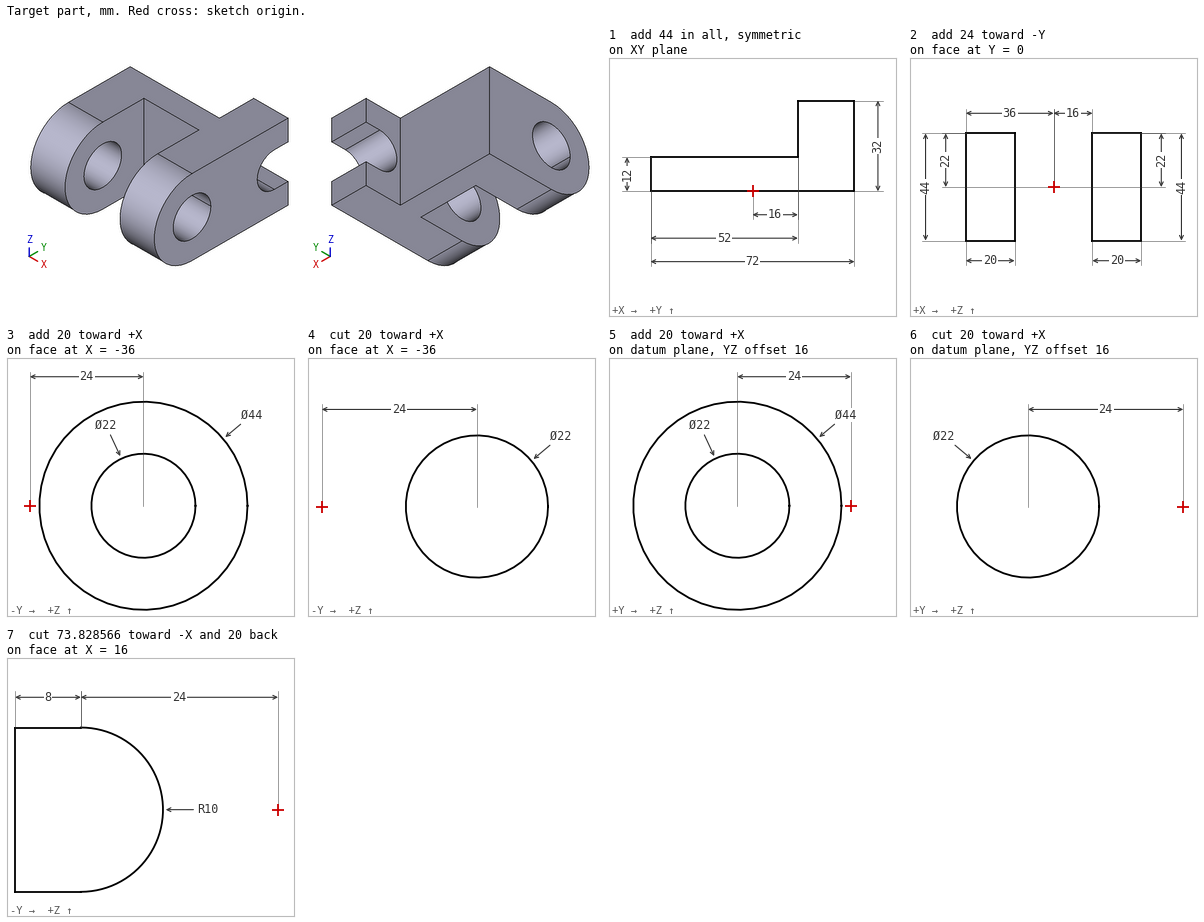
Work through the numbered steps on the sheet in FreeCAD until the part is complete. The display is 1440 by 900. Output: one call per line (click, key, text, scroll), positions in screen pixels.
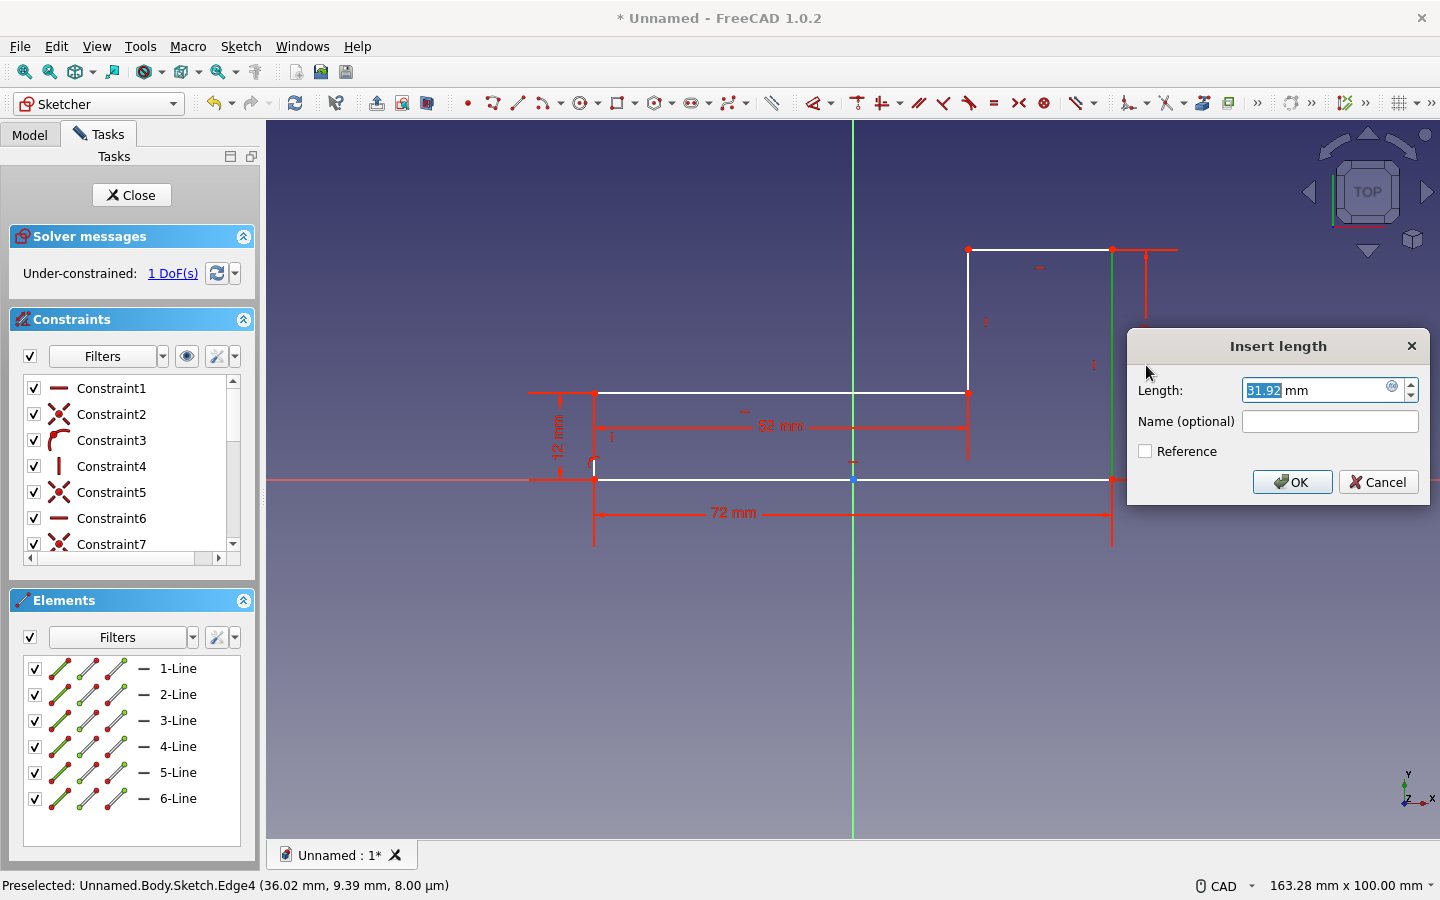
text(32)
key(Return)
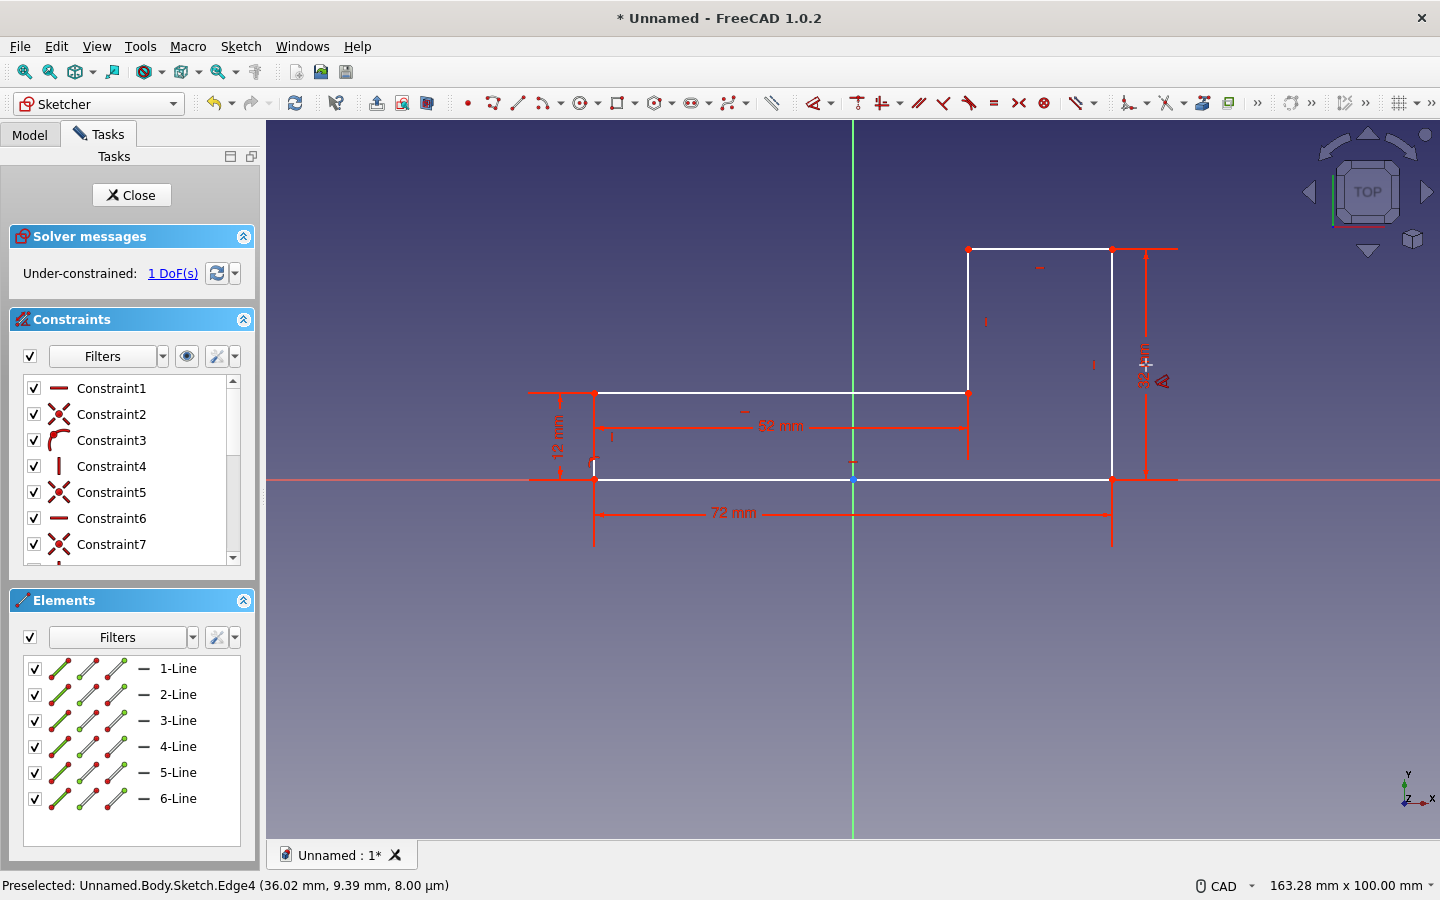
click(968, 393)
click(911, 514)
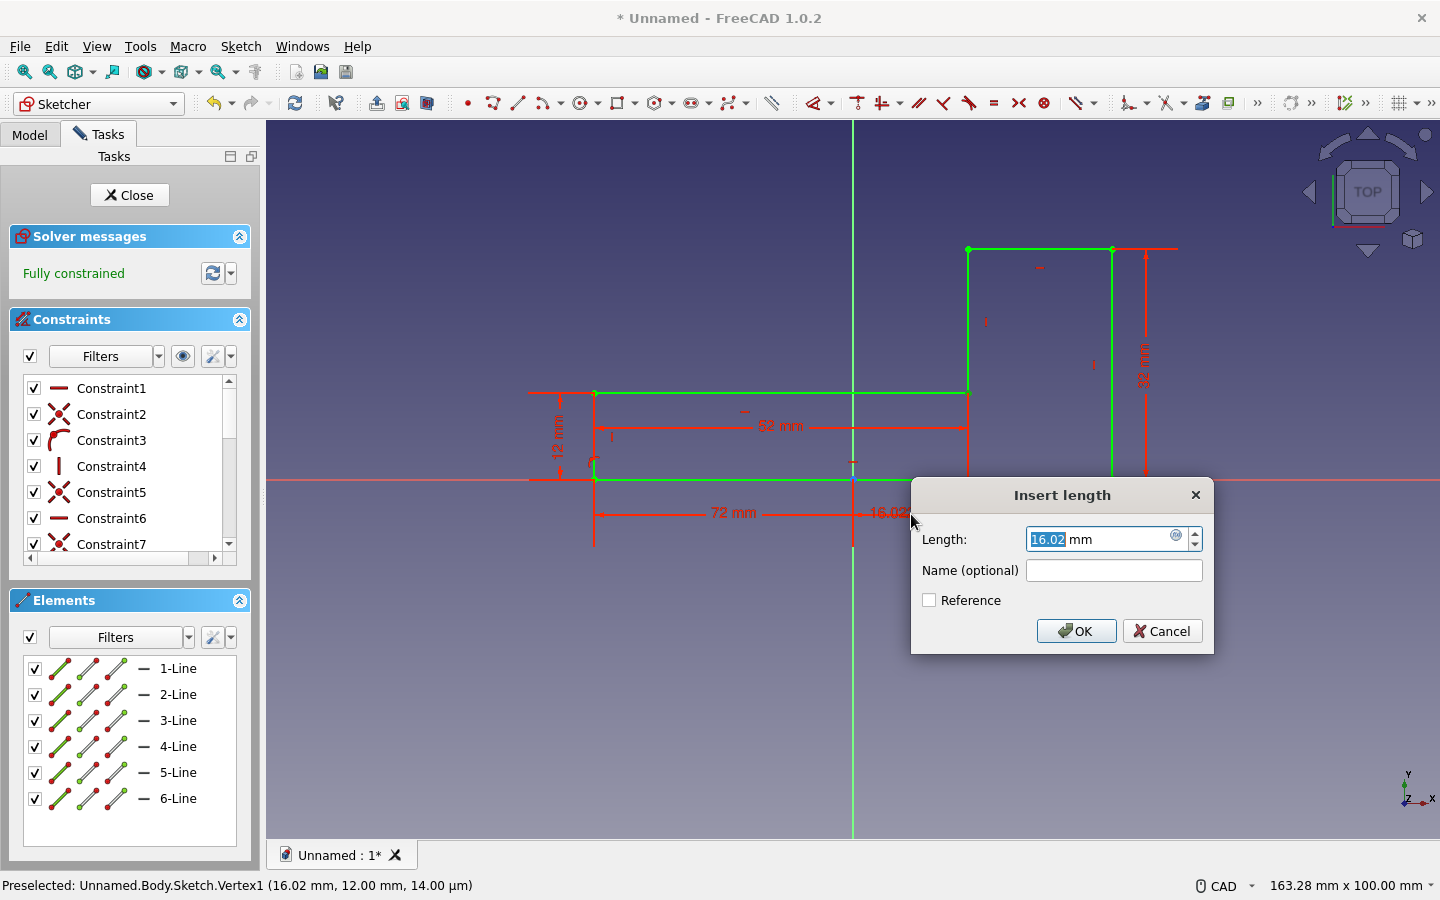
text(16)
key(Return)
key(Escape)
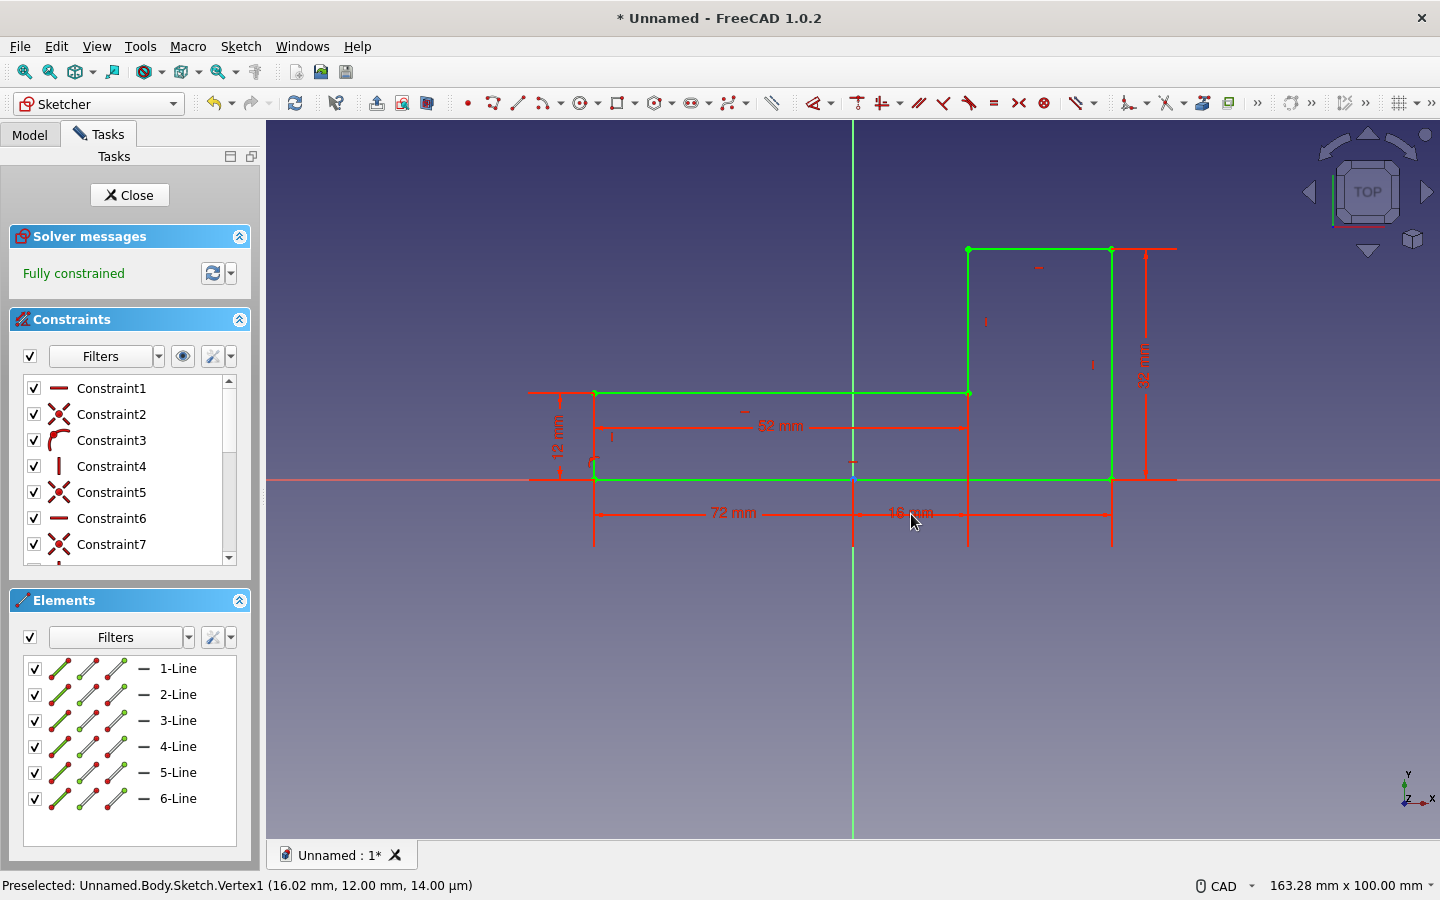
click(130, 195)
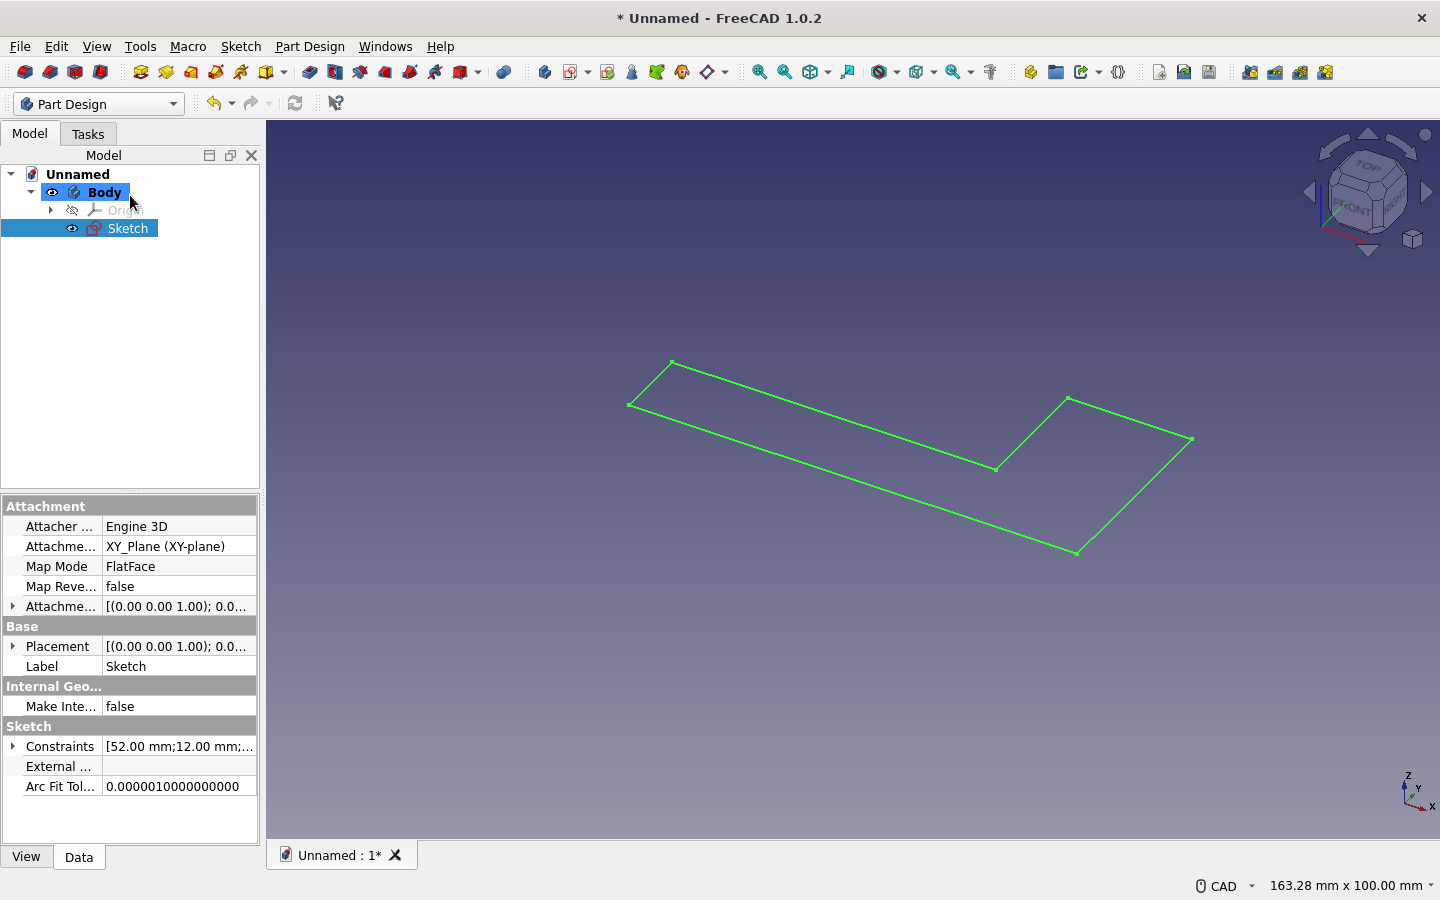
click(141, 72)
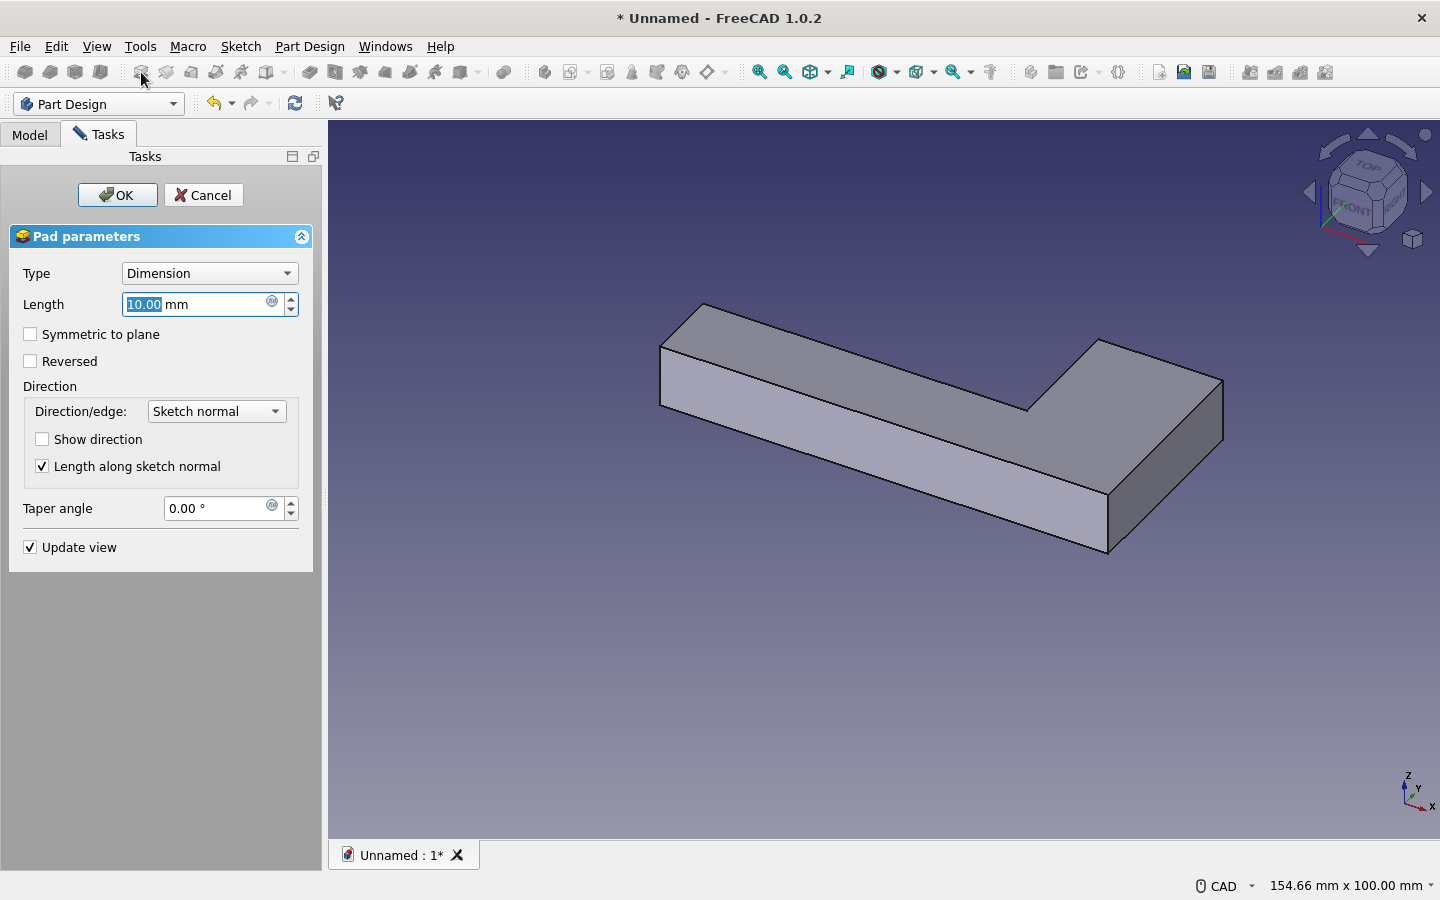
text(44)
key(Tab)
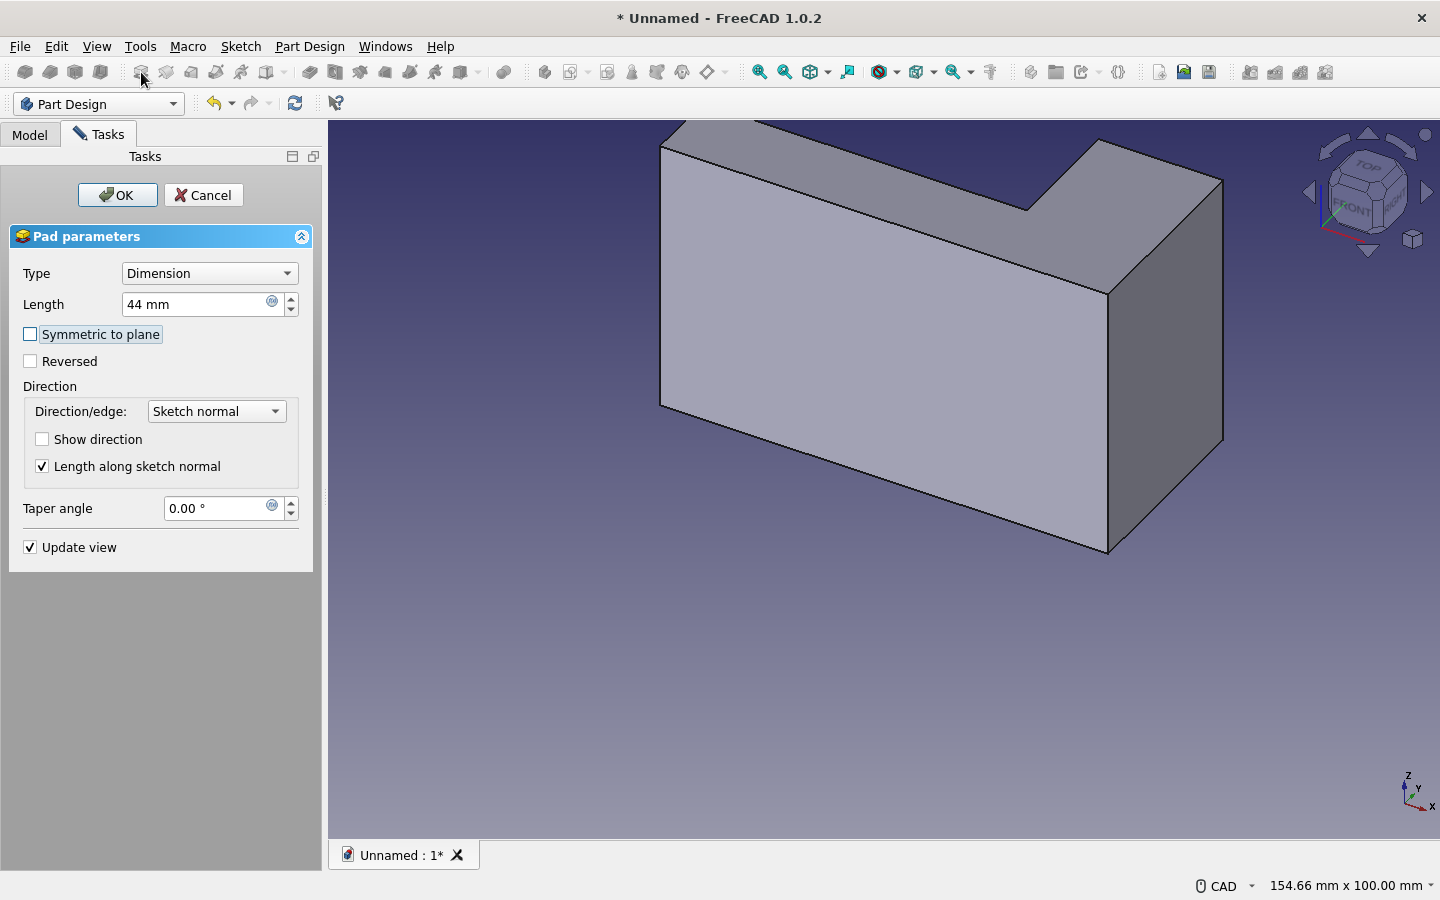
click(31, 334)